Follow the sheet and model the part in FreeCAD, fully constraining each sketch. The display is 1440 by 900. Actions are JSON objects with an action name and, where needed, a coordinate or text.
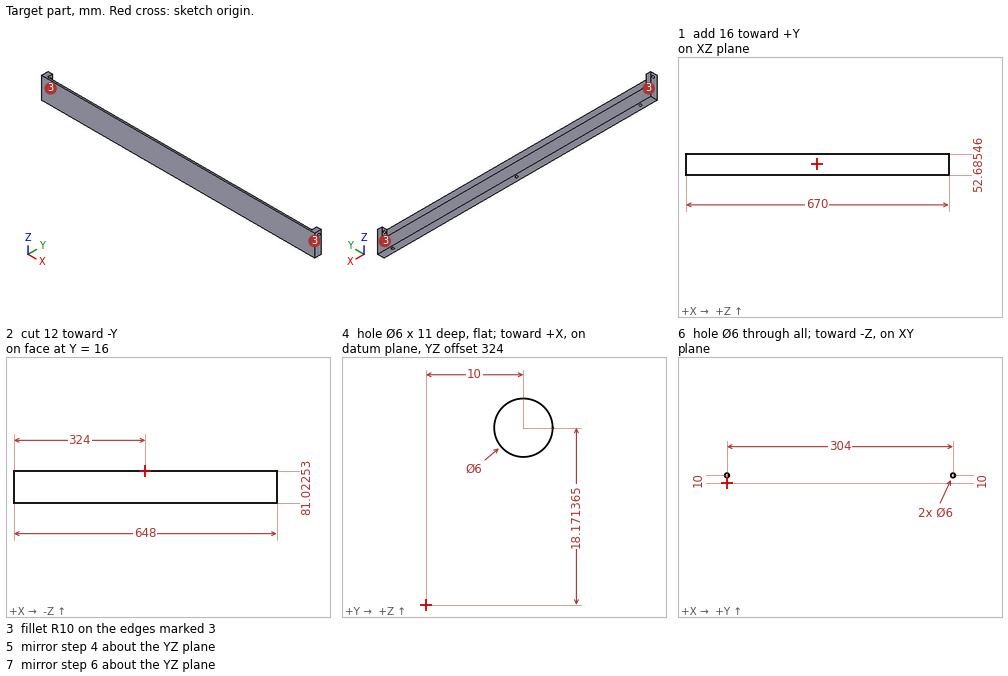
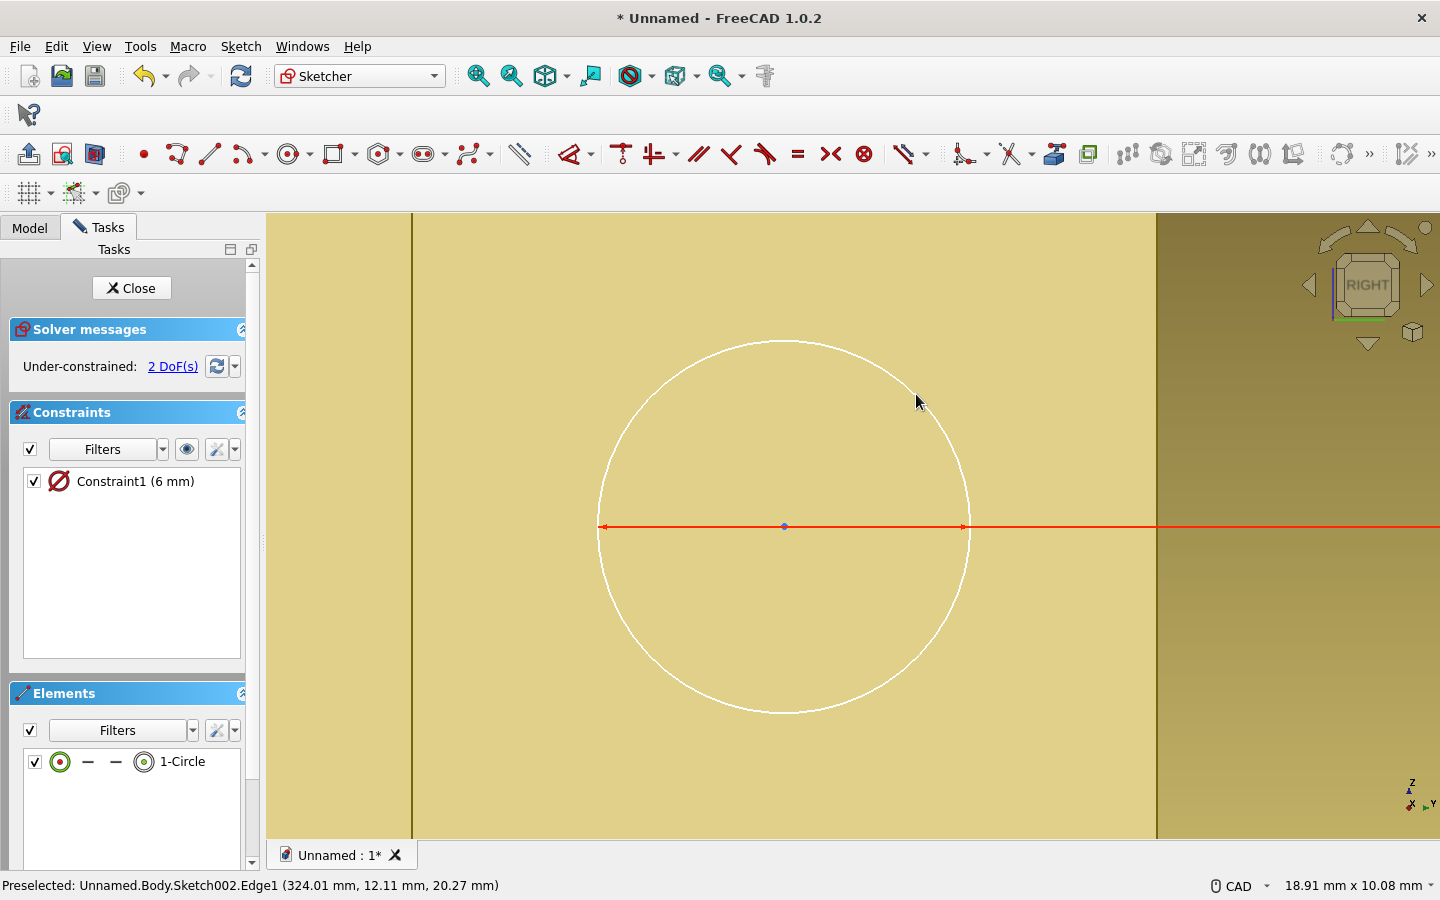
{"action": "left_click", "coordinate": [784, 527]}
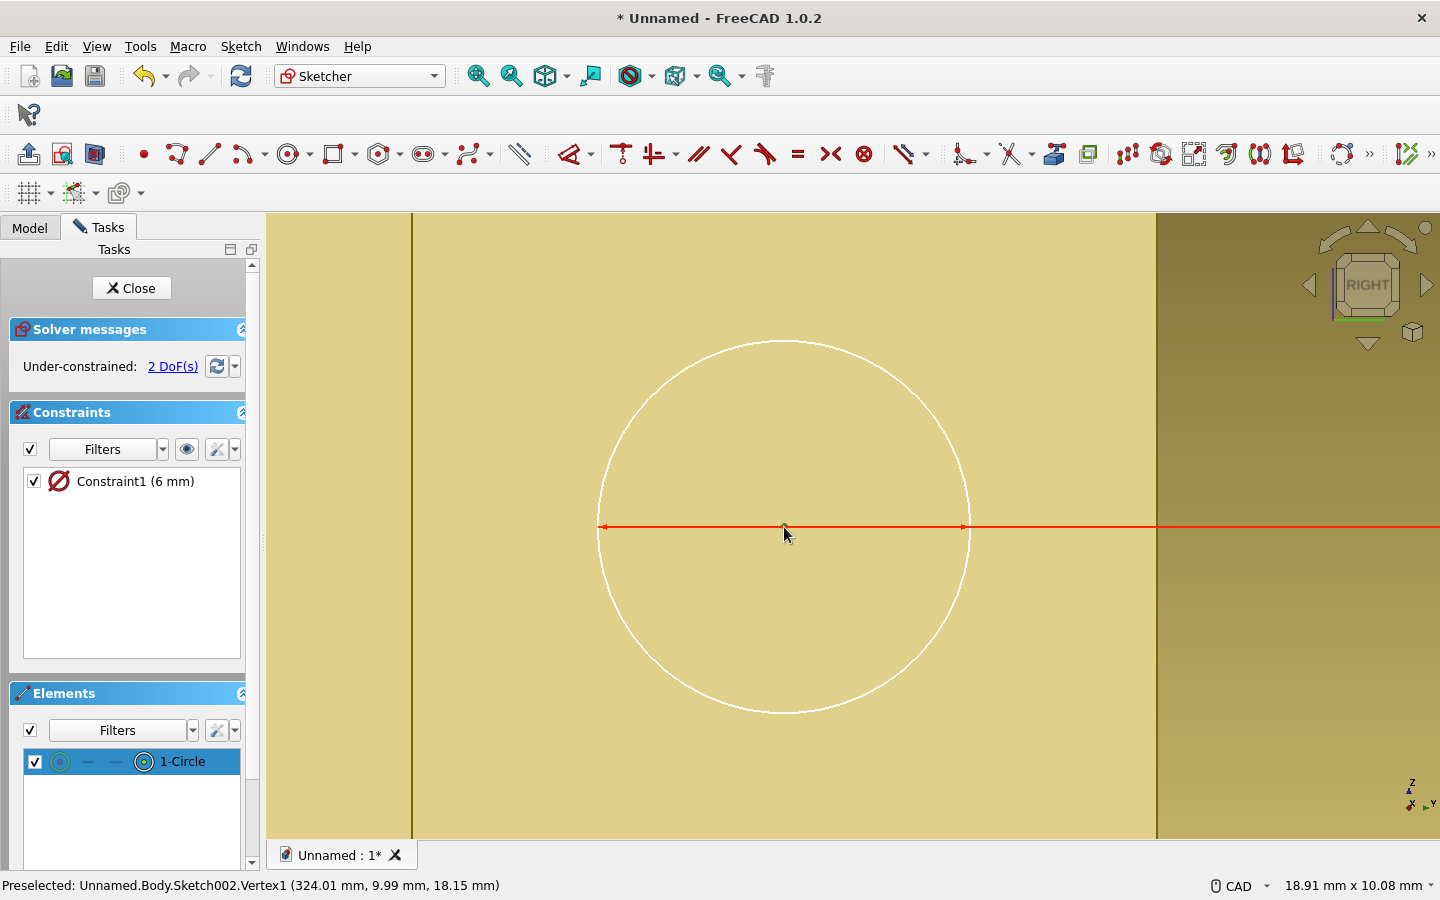
{"action": "left_click", "coordinate": [590, 154]}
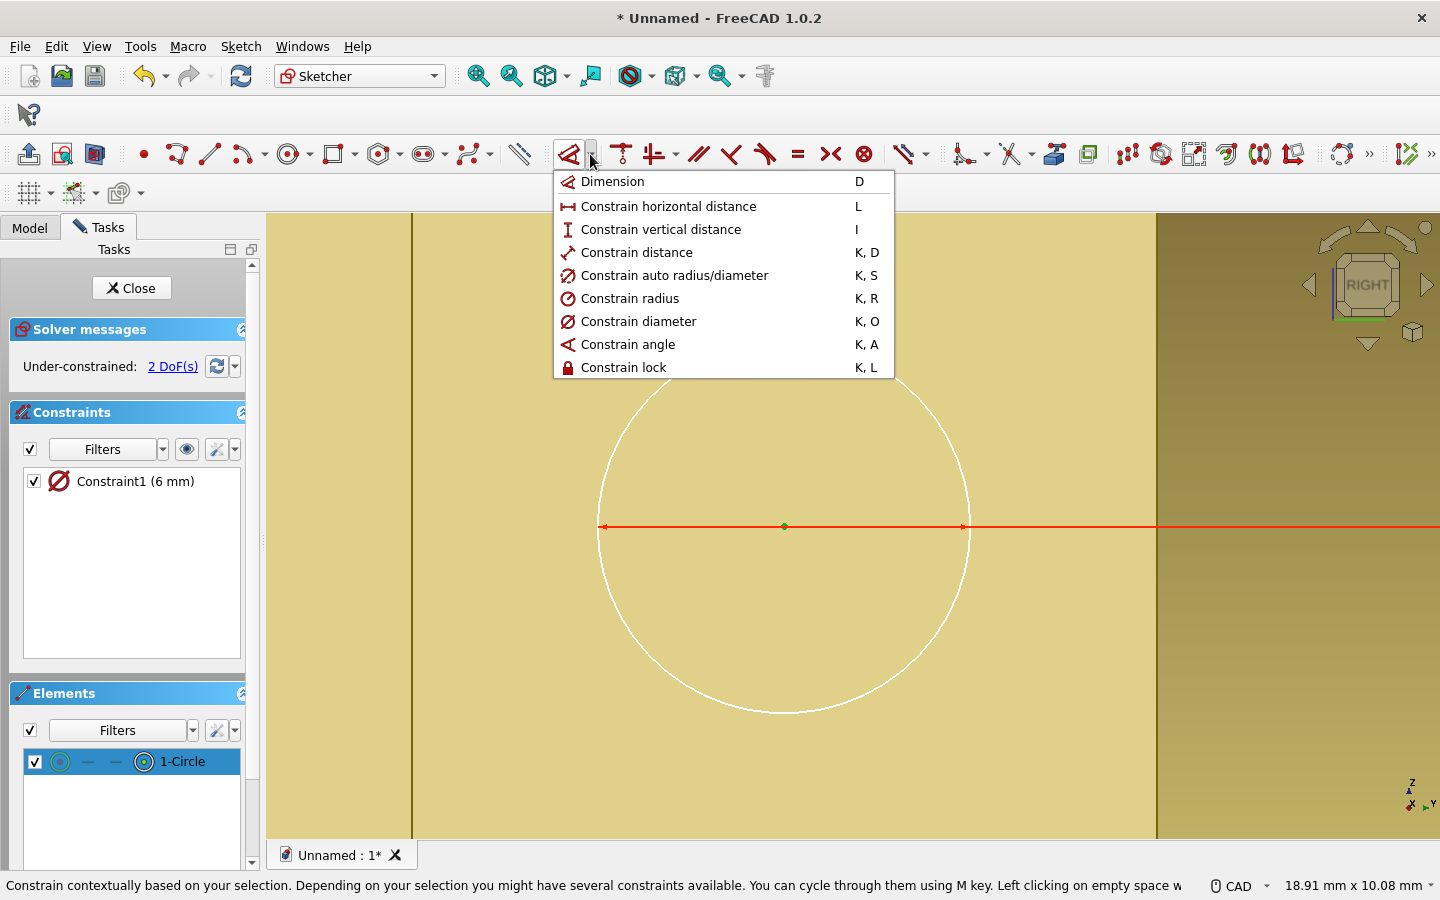
{"action": "left_click", "coordinate": [724, 206]}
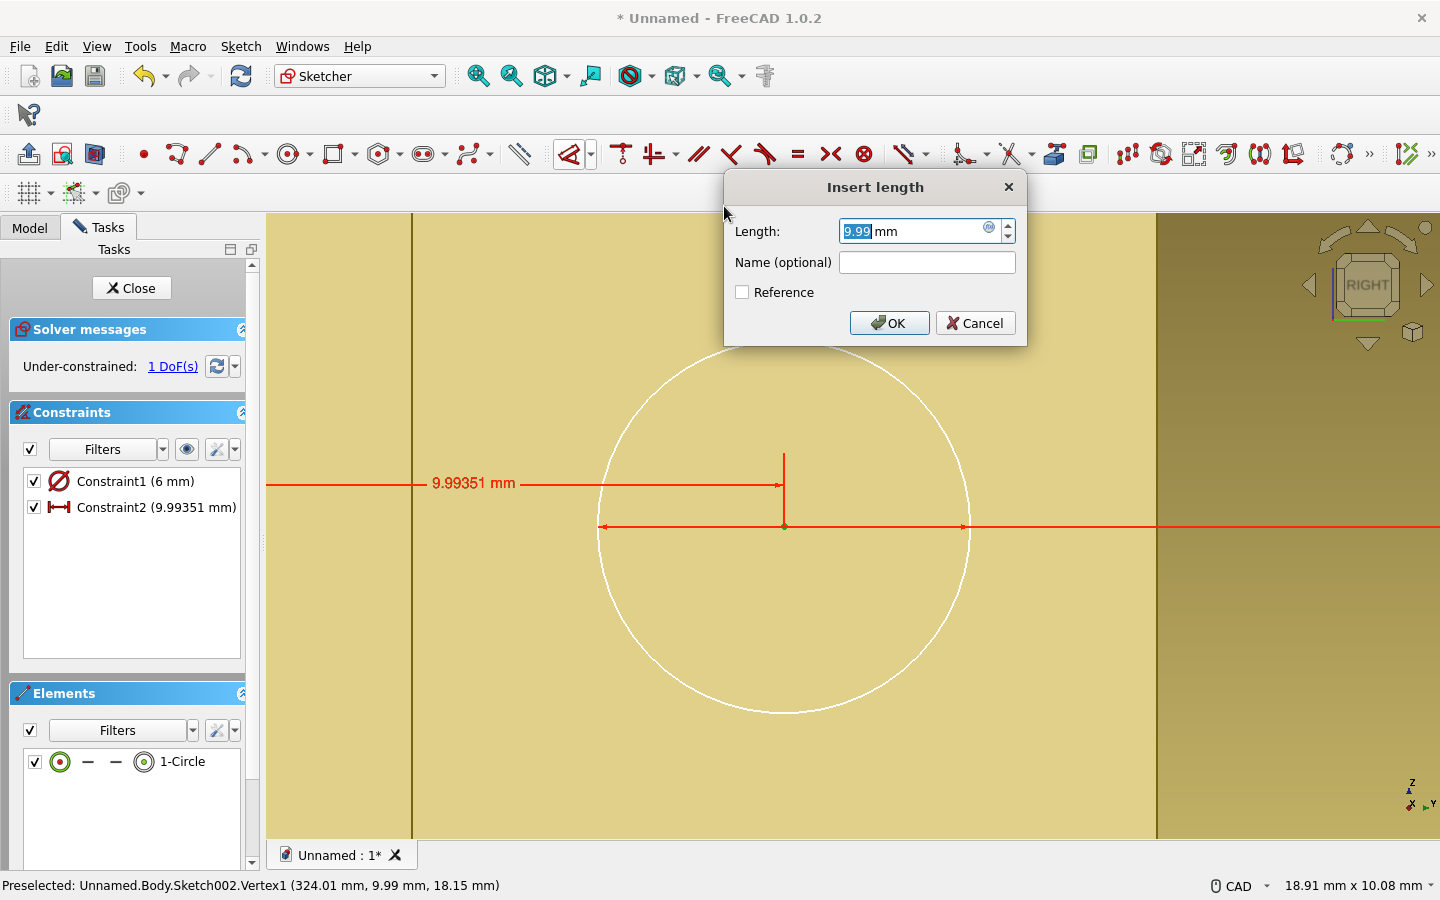
{"action": "type", "text": "10"}
{"action": "key", "text": "Return"}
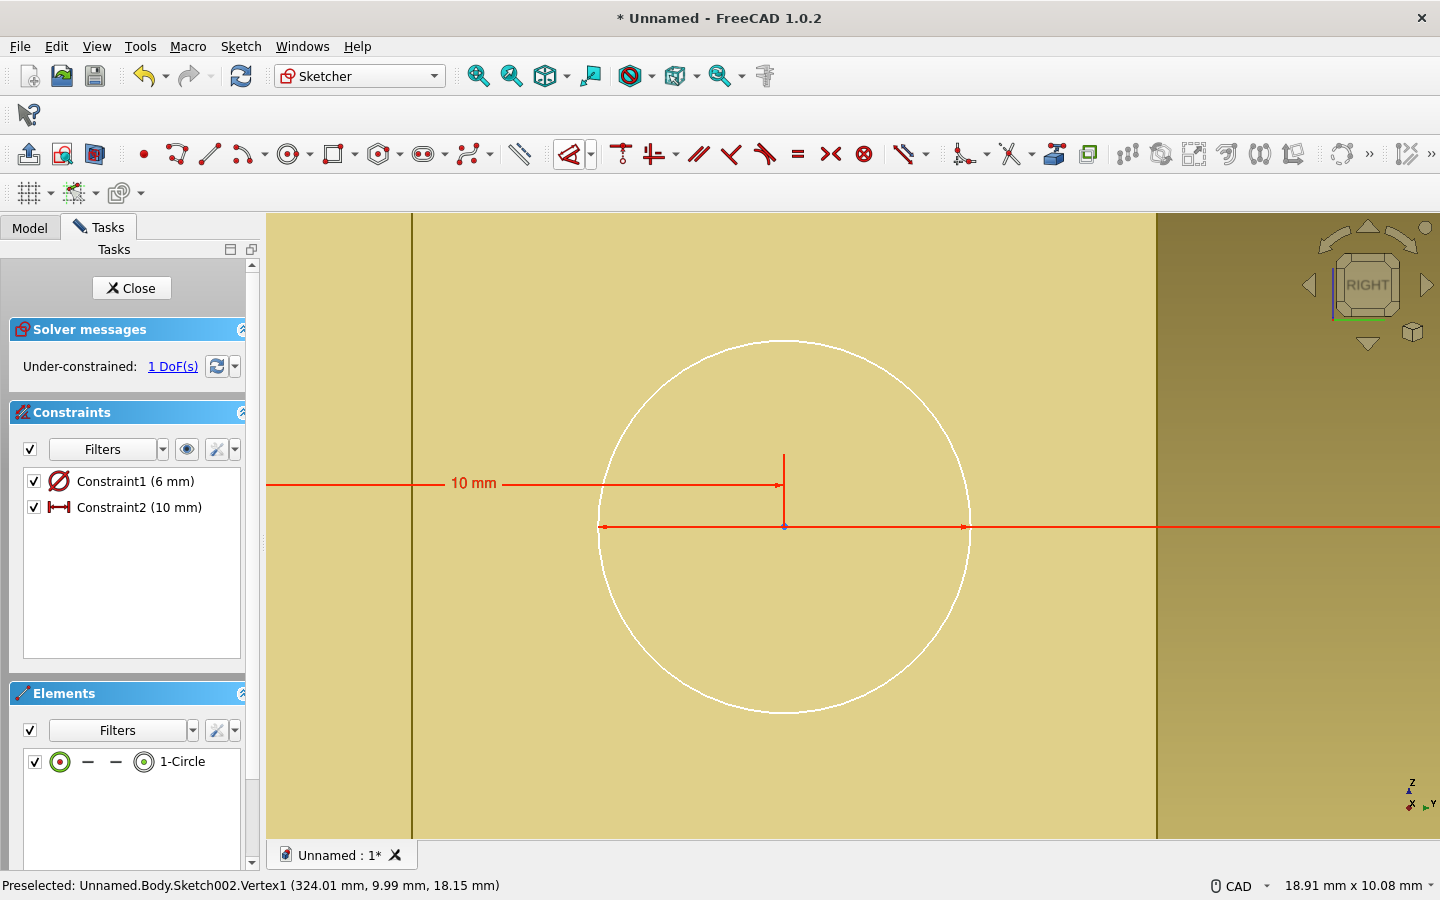
{"action": "left_click", "coordinate": [784, 527]}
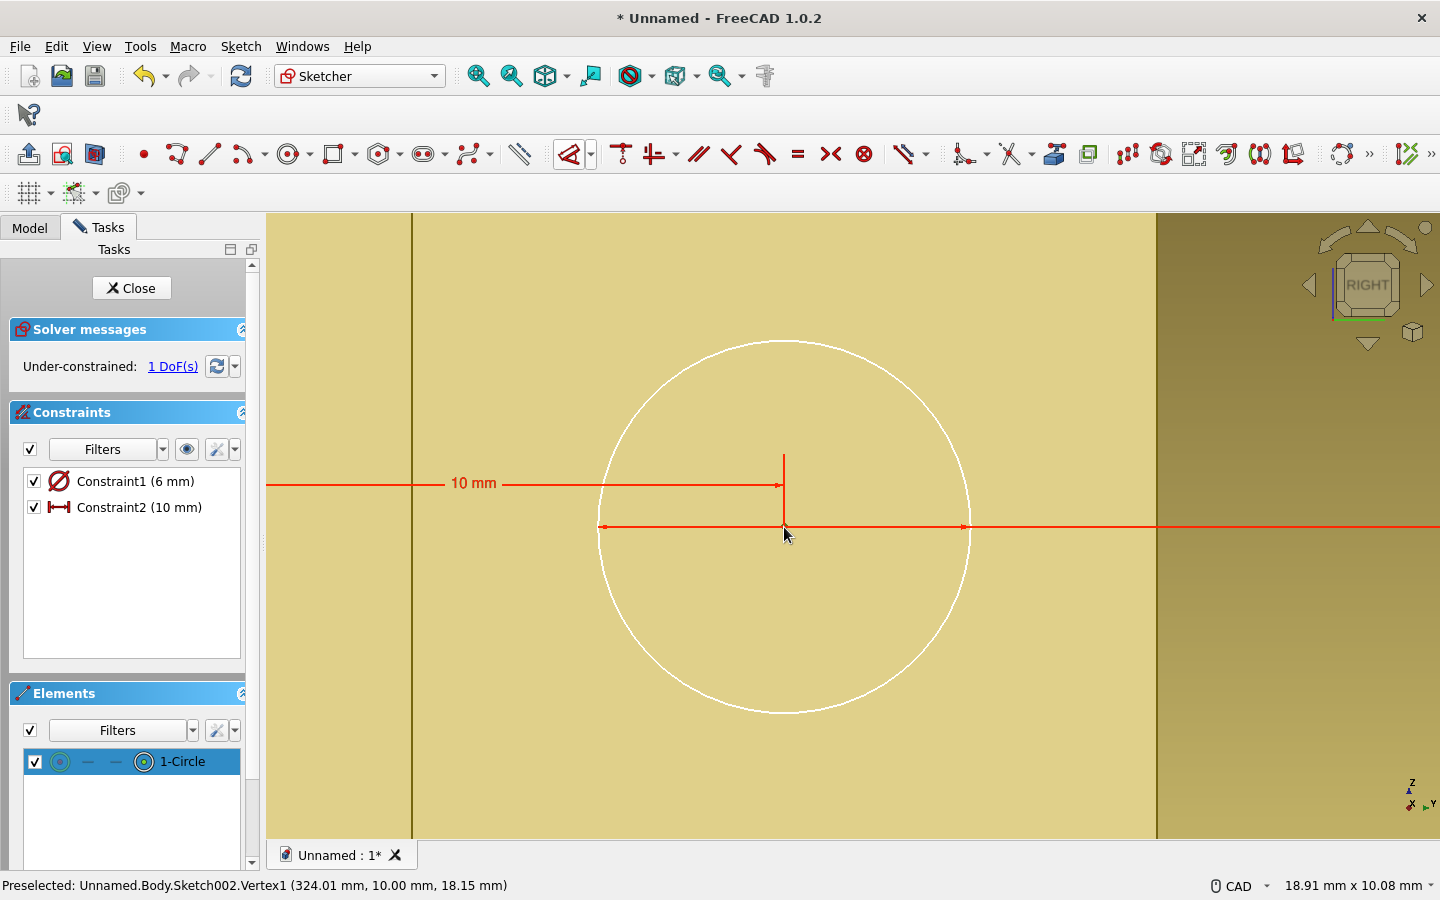
{"action": "left_click", "coordinate": [590, 154]}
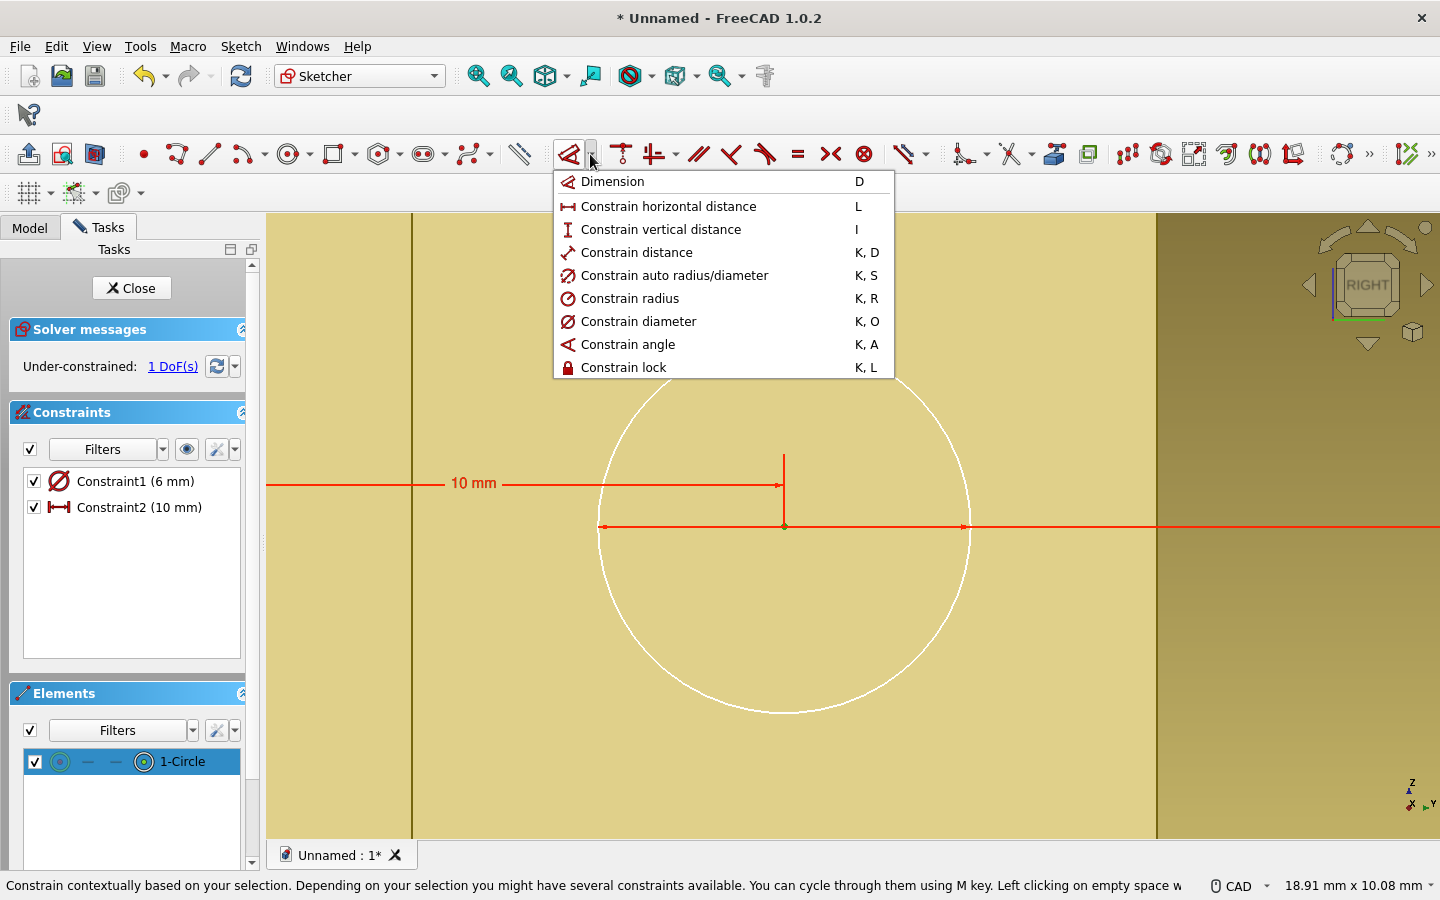
{"action": "left_click", "coordinate": [724, 230]}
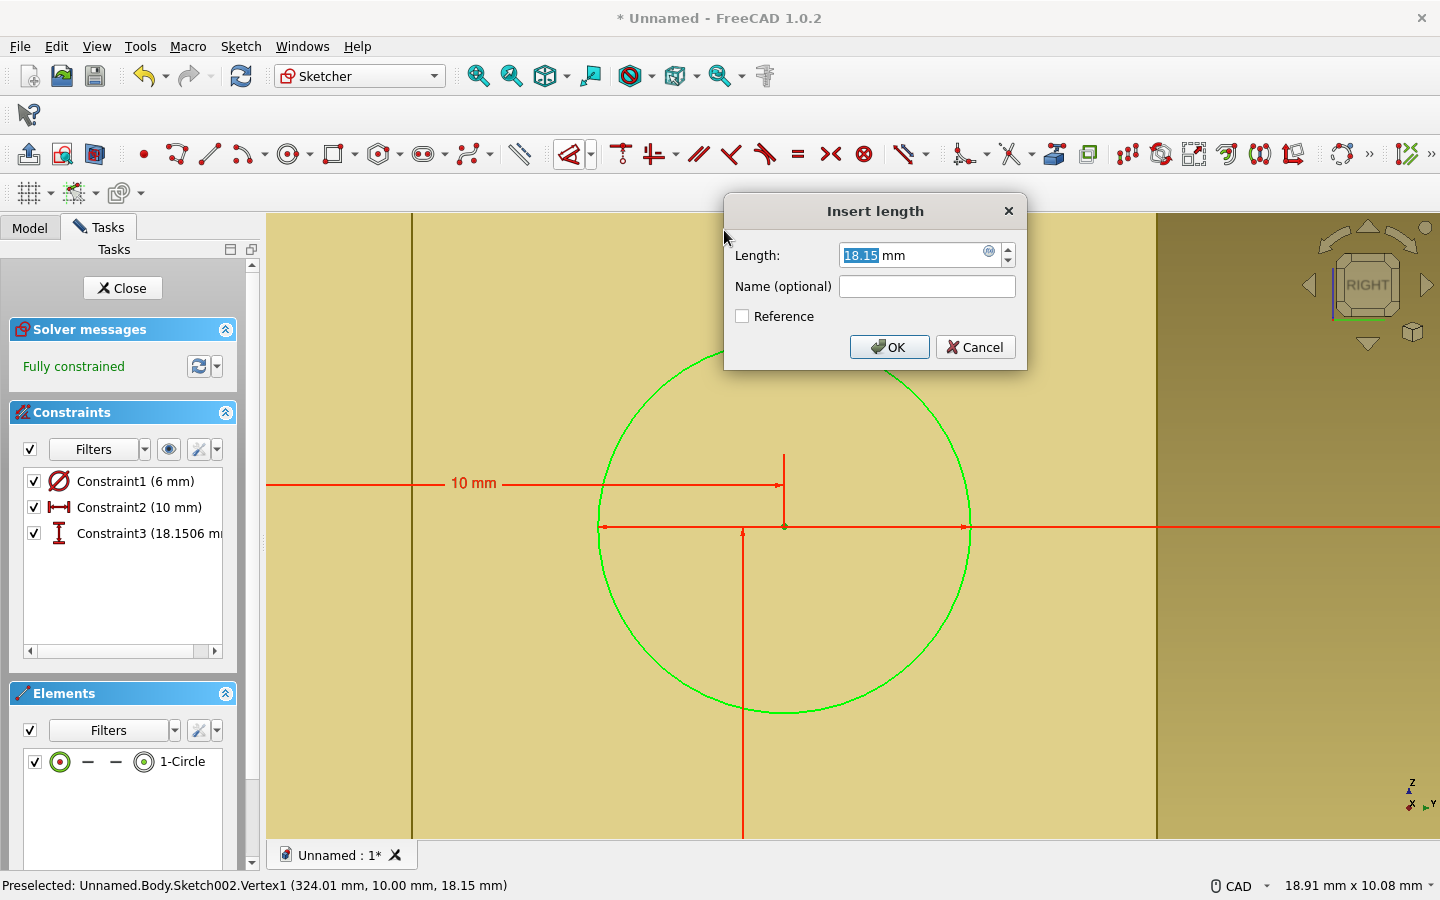
{"action": "type", "text": "18.171365"}
{"action": "key", "text": "Return"}